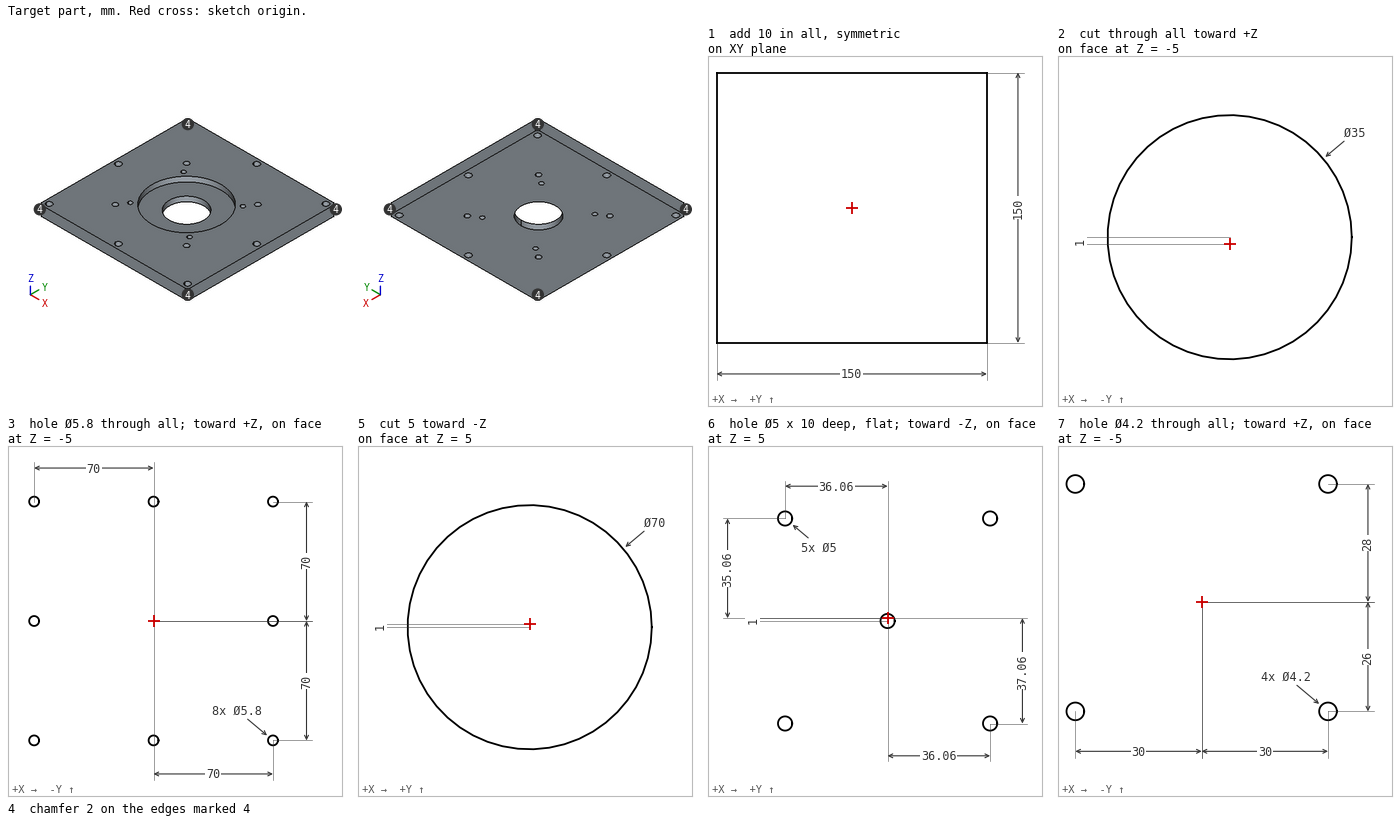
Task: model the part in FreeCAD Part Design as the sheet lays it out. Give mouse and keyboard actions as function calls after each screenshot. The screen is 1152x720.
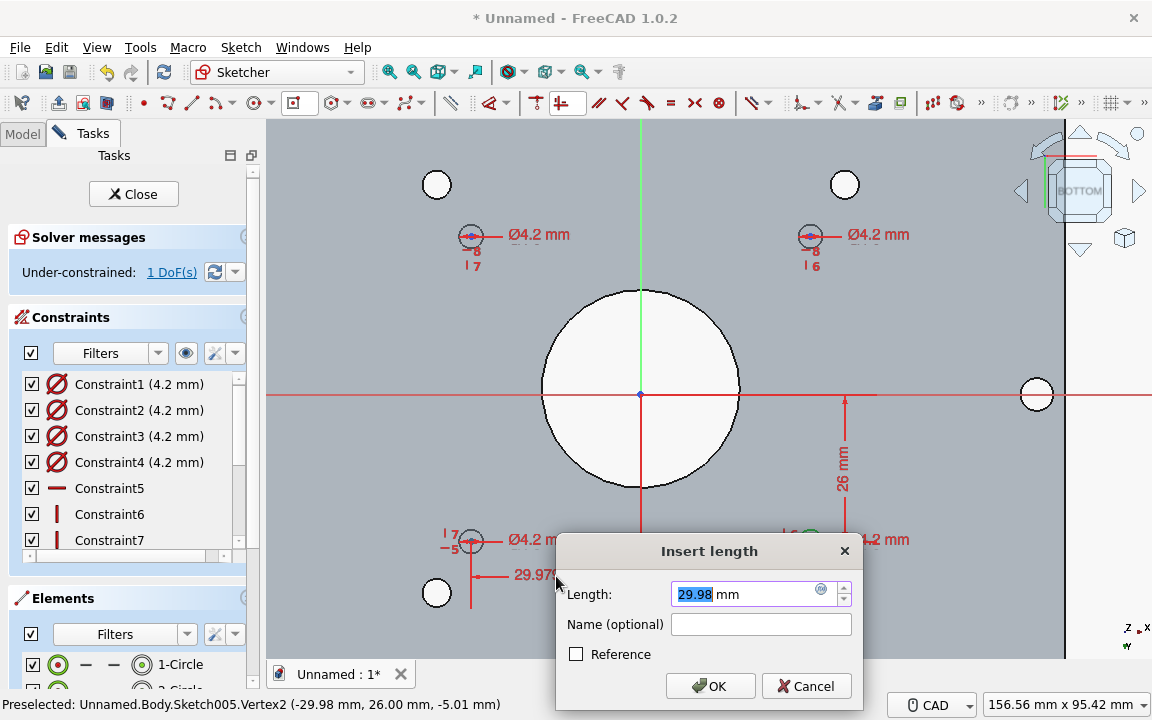
text(30)
key(Return)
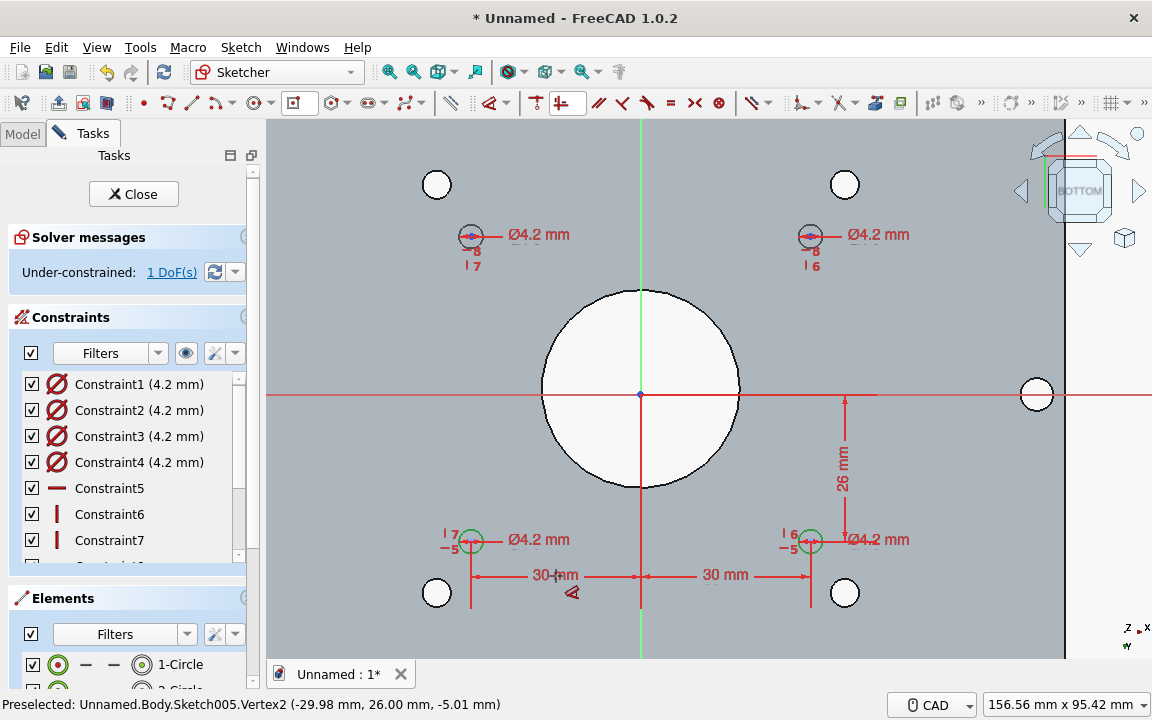
click(811, 237)
click(845, 316)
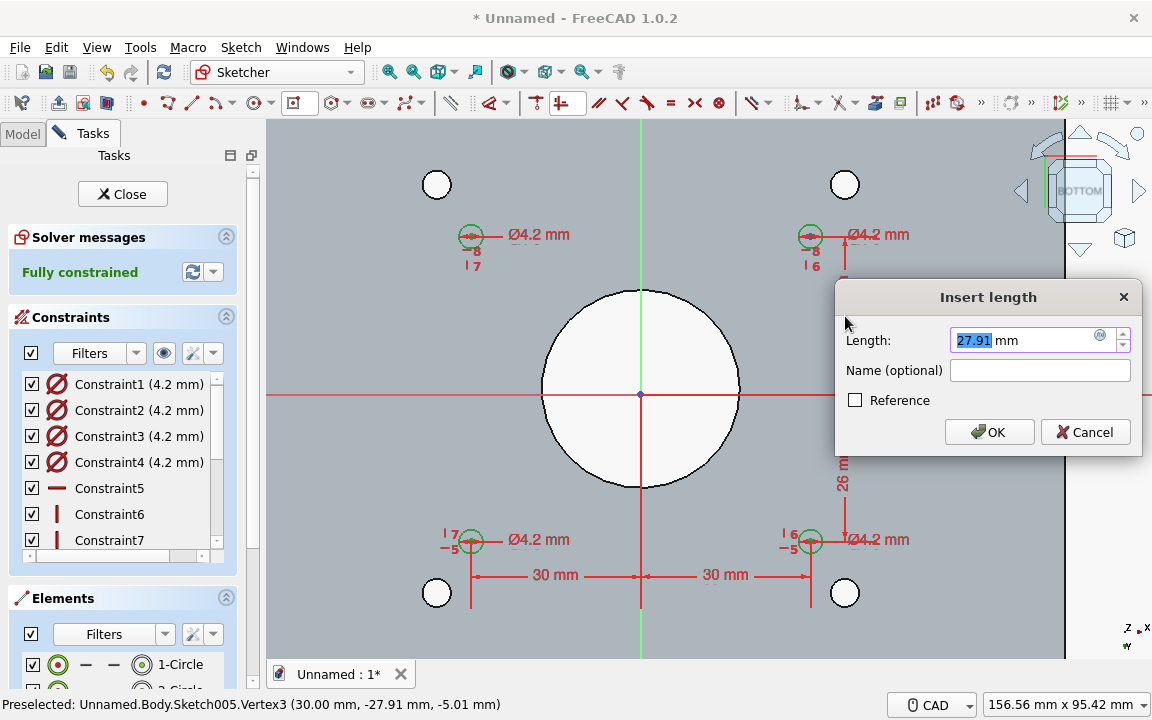
text(28)
key(Return)
key(Escape)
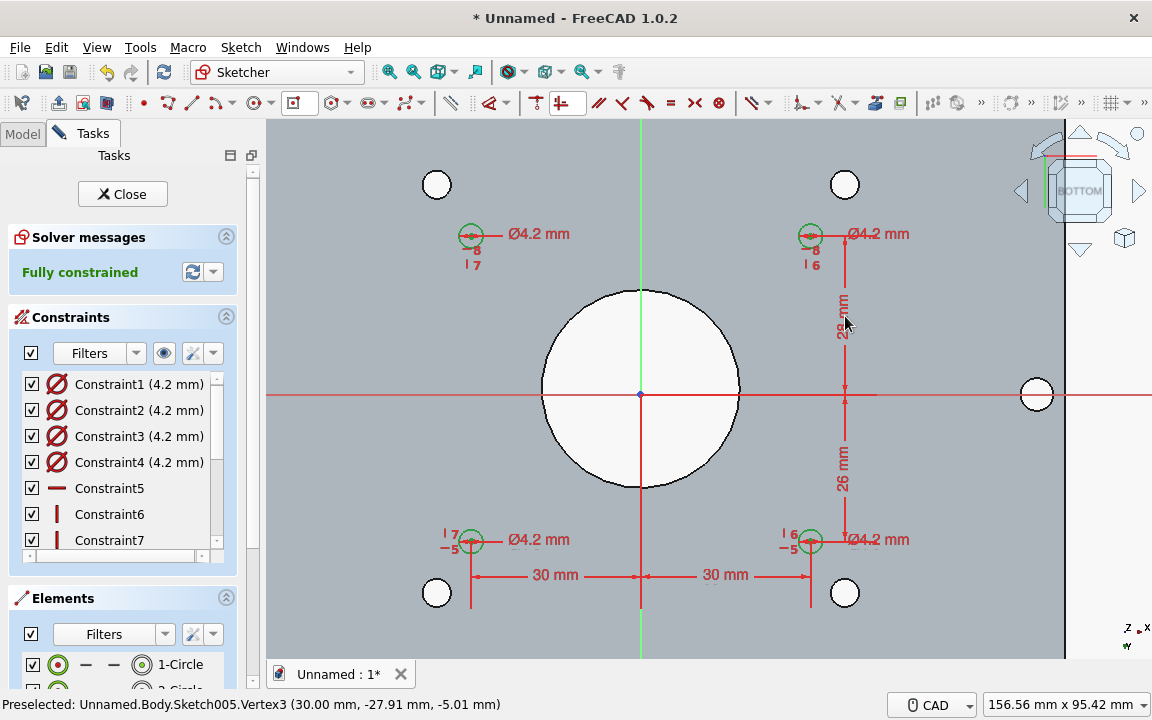
click(123, 194)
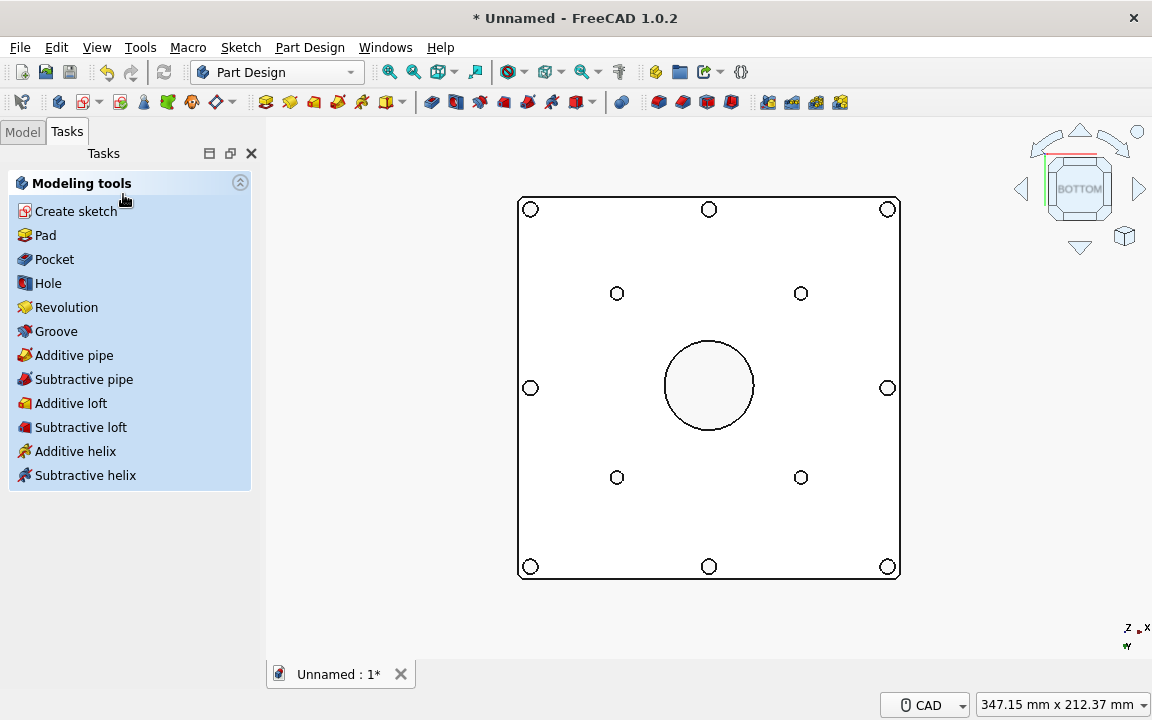
click(456, 102)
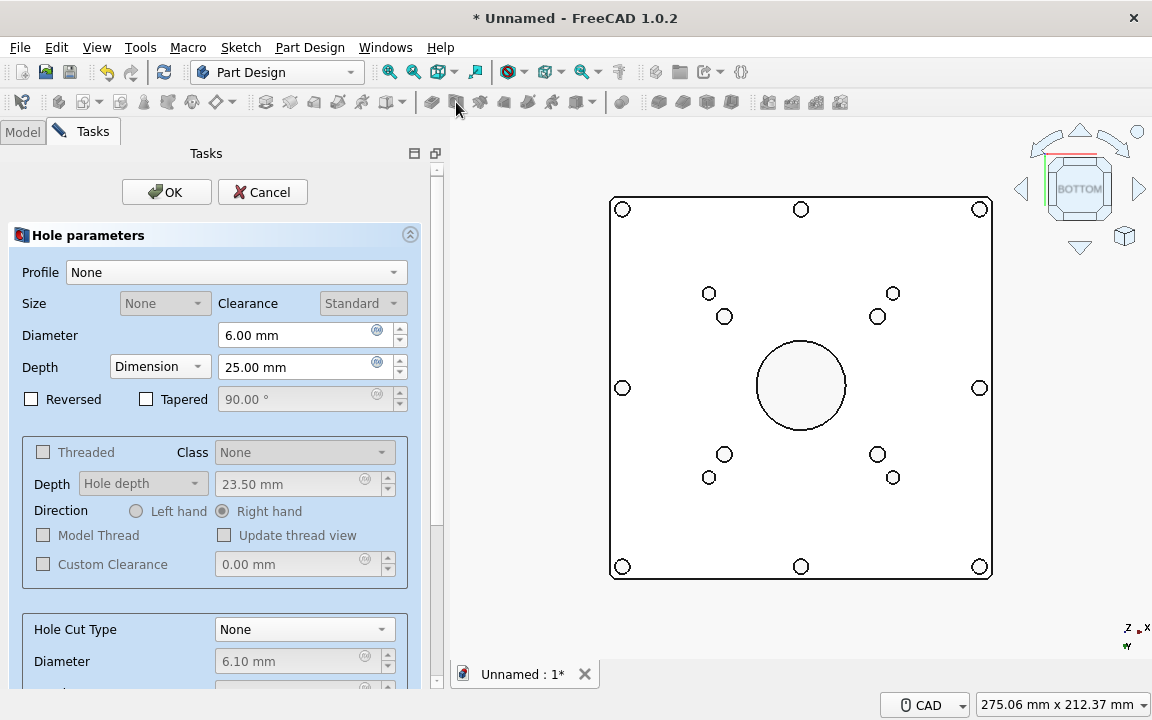
triple_click(305, 335)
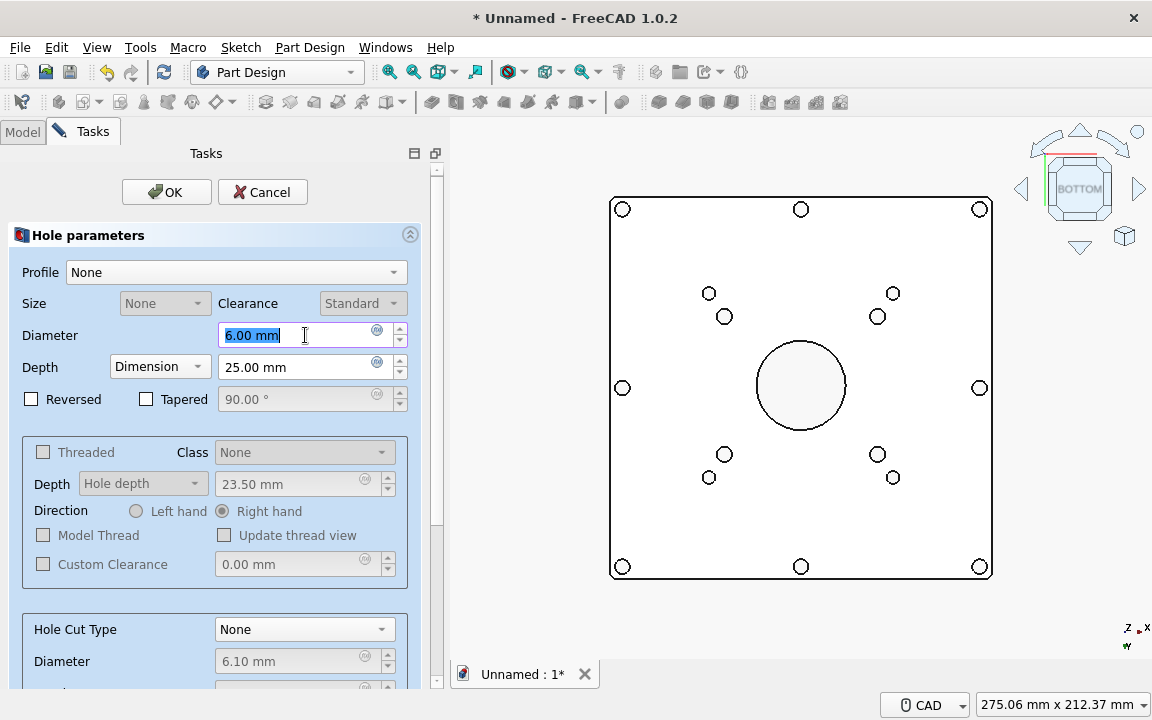
text(4.2)
key(Tab)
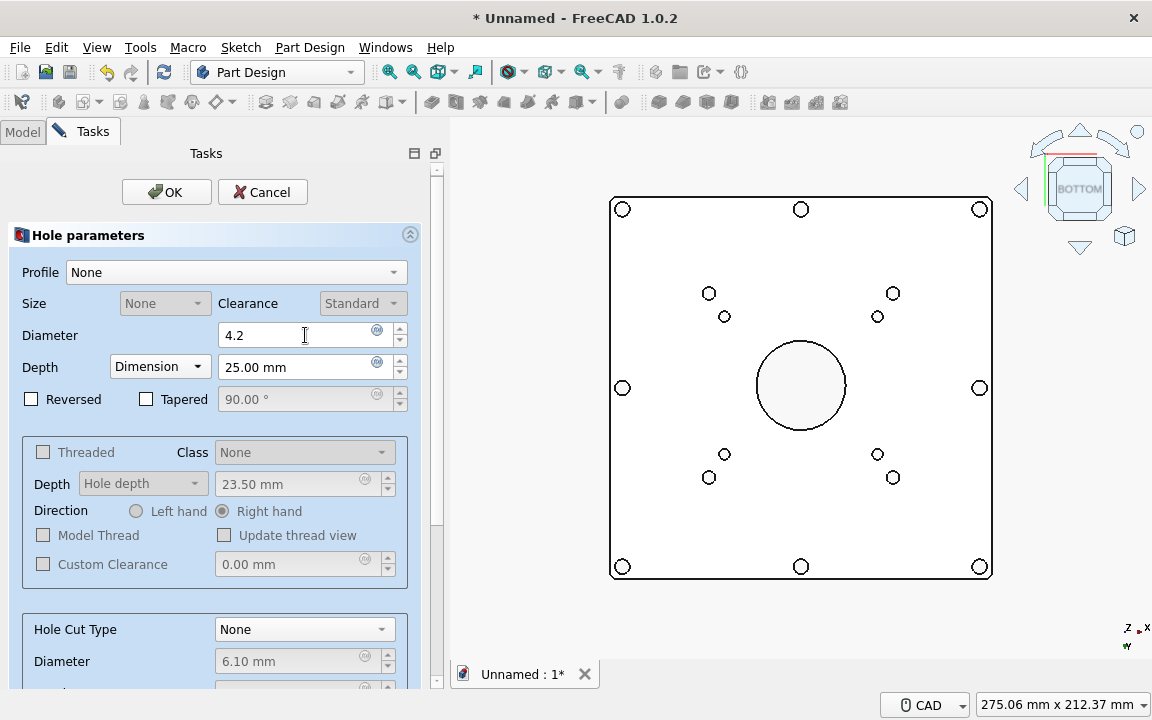
click(161, 366)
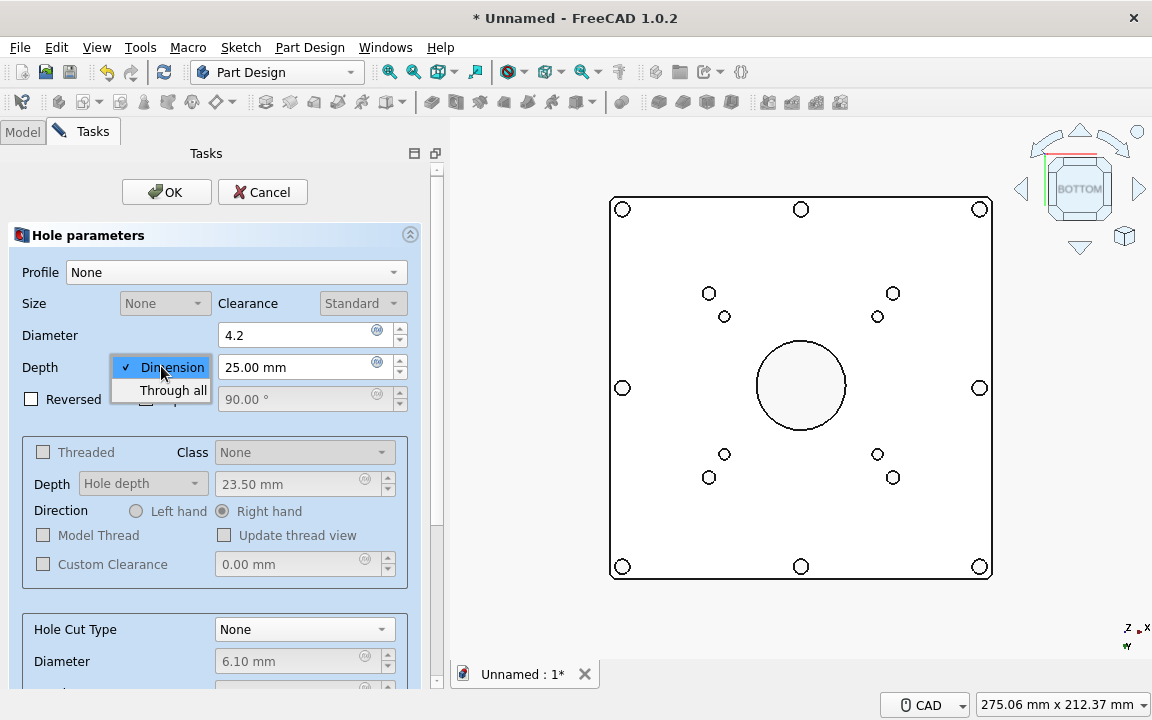
click(160, 390)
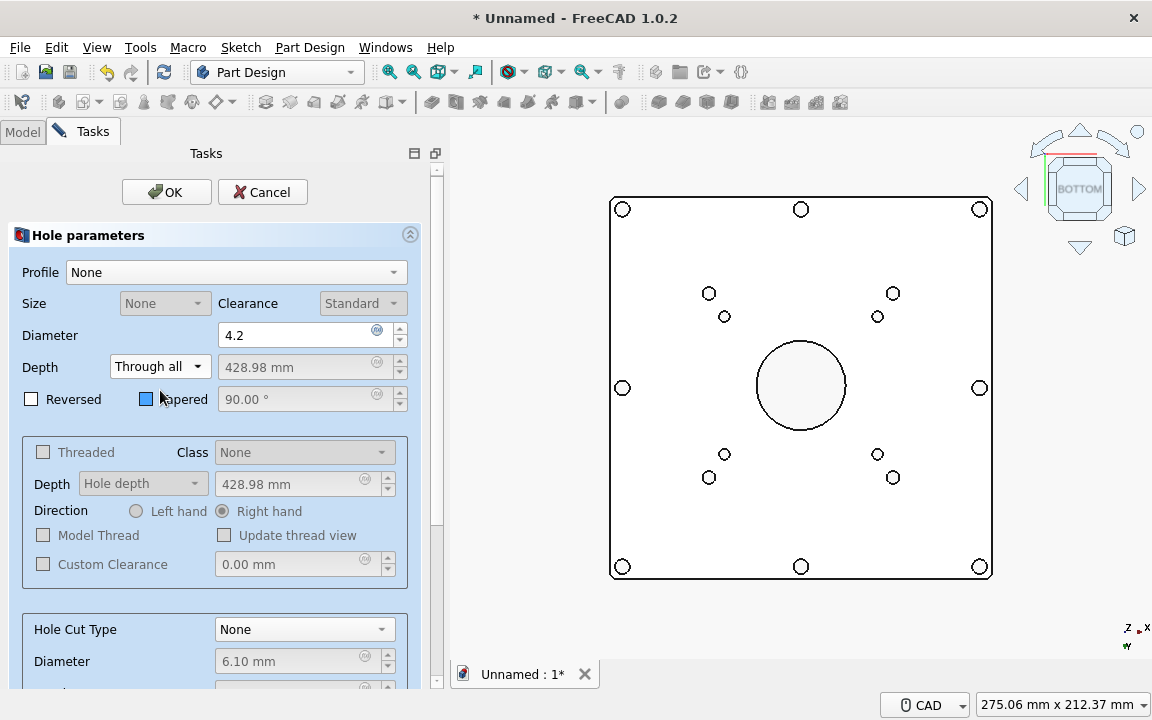
click(167, 192)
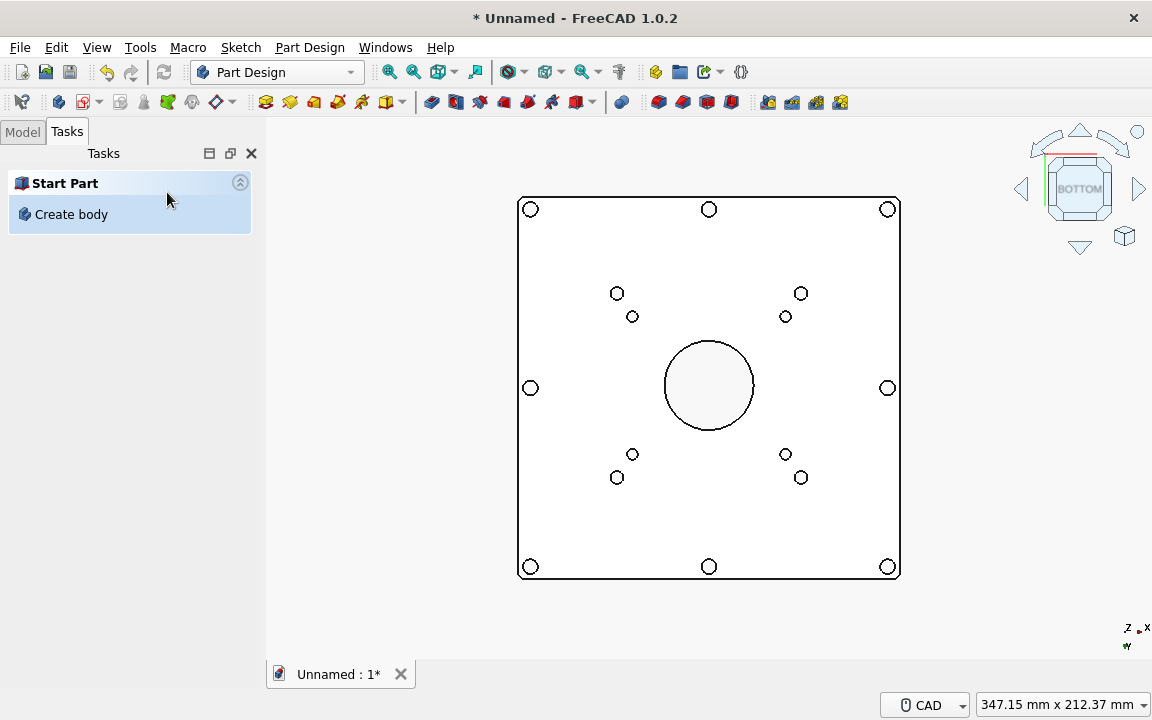
key(0)